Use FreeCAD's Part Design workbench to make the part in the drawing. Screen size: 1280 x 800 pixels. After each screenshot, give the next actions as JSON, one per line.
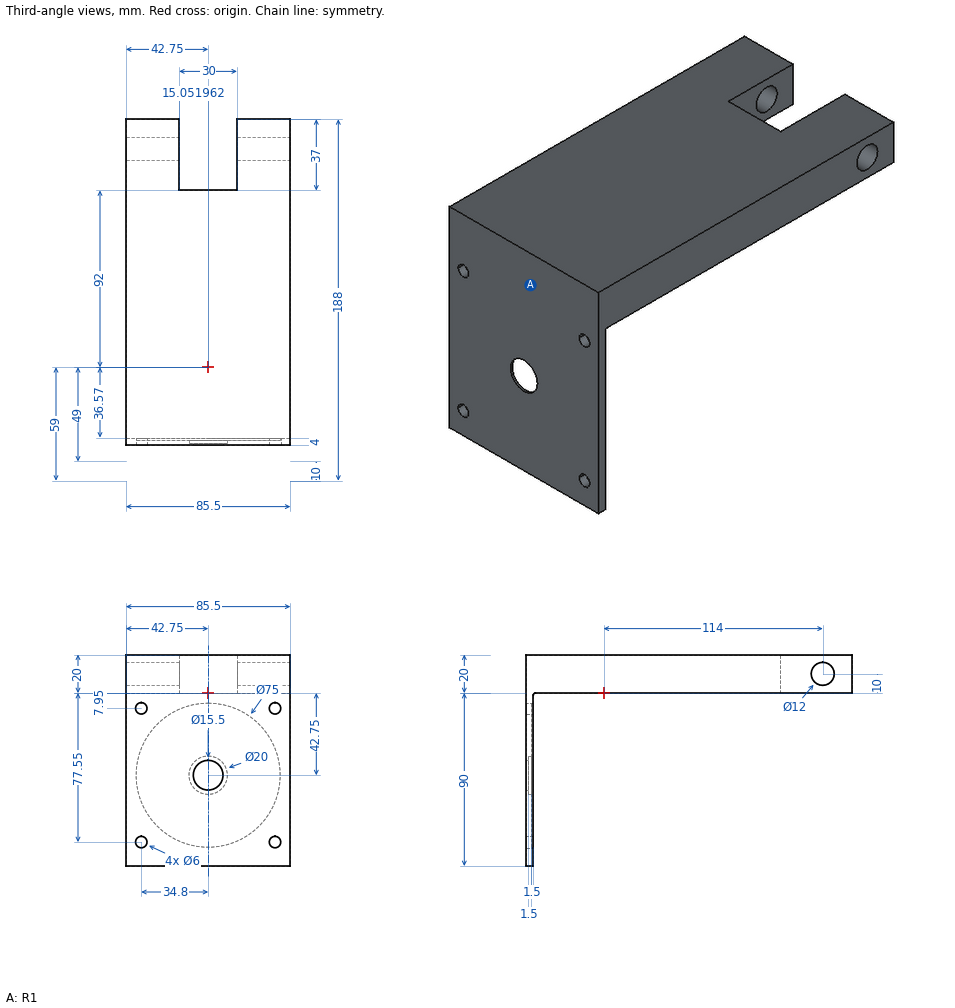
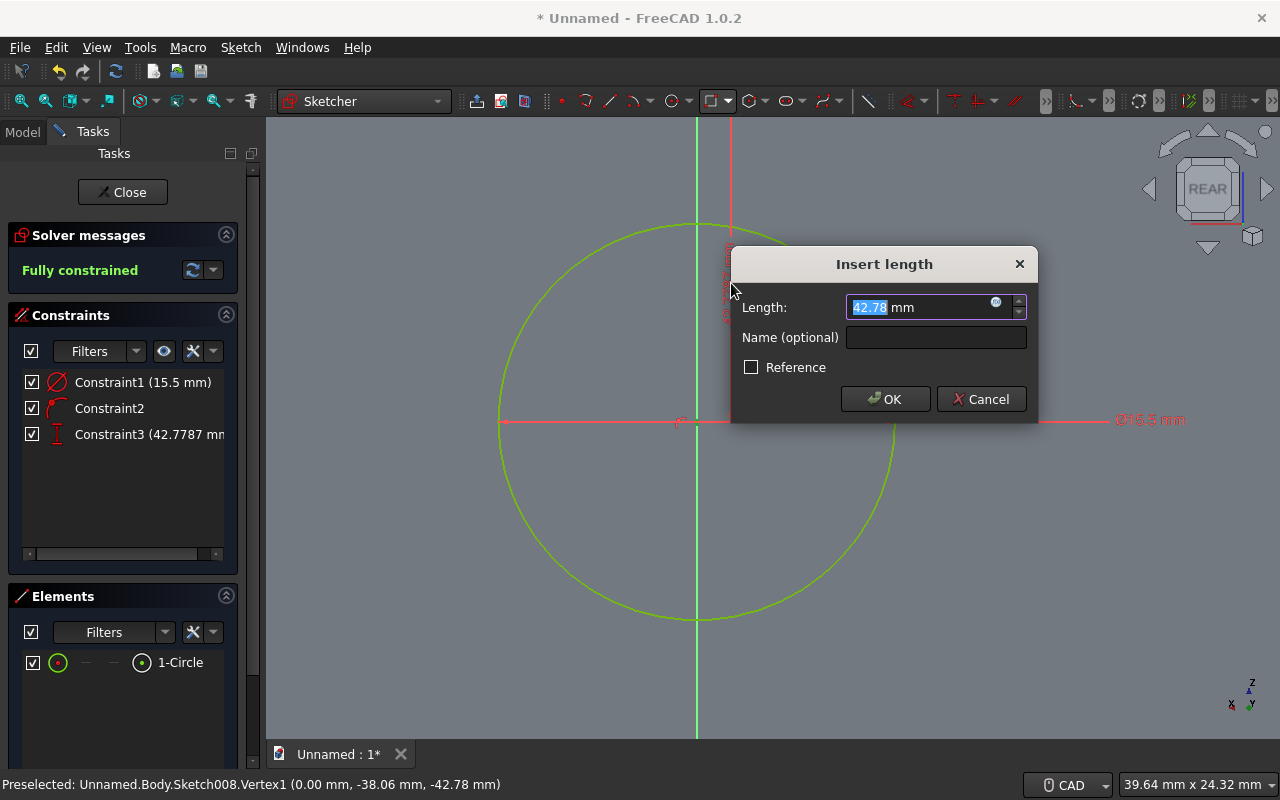
{"action": "type", "text": "42.75"}
{"action": "key", "text": "Return"}
{"action": "key", "text": "Escape"}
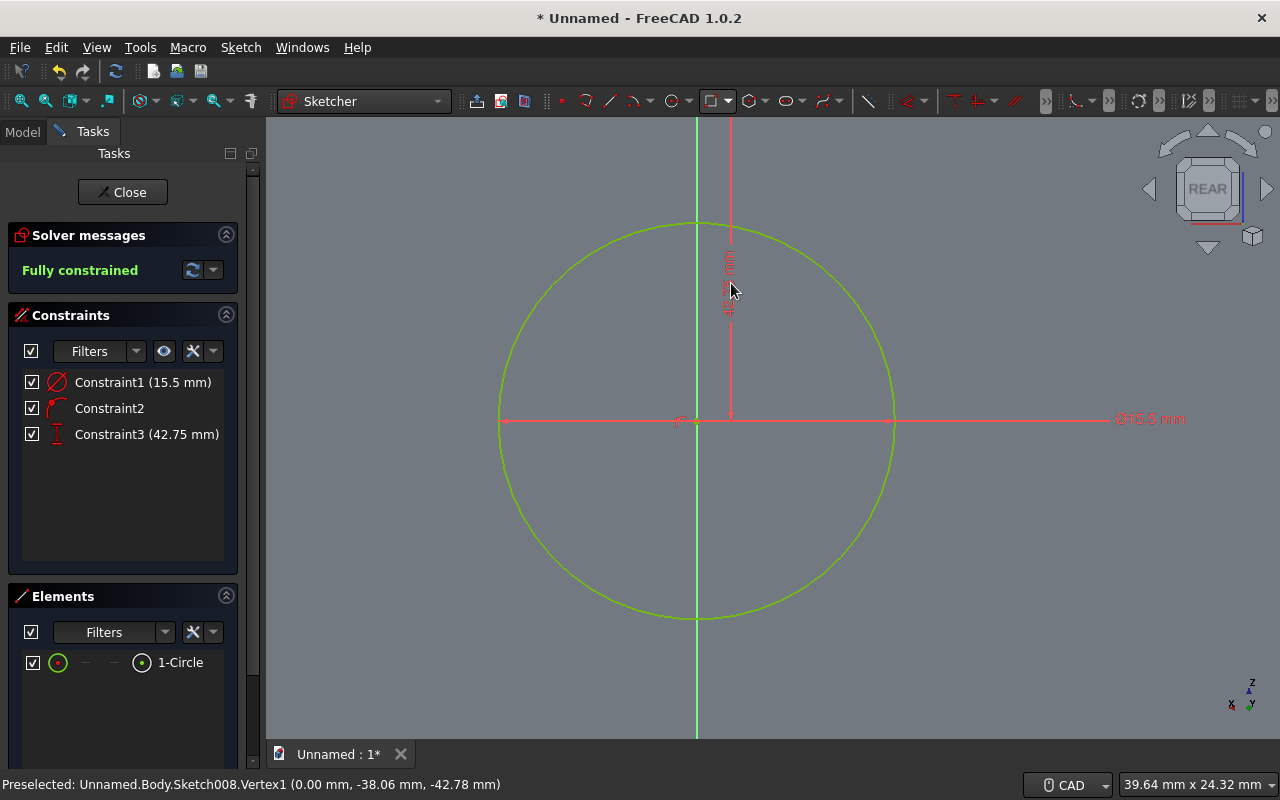
{"action": "left_click", "coordinate": [123, 192]}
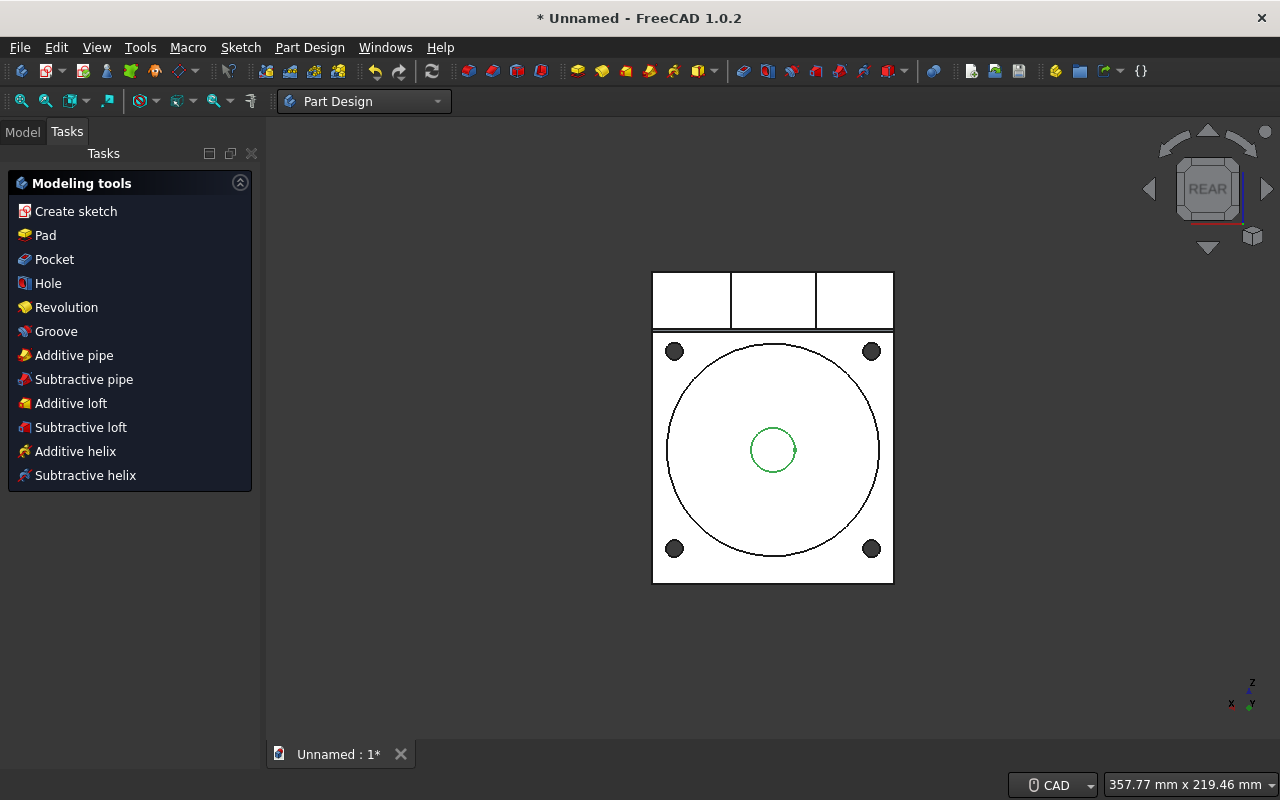
{"action": "left_click", "coordinate": [744, 72]}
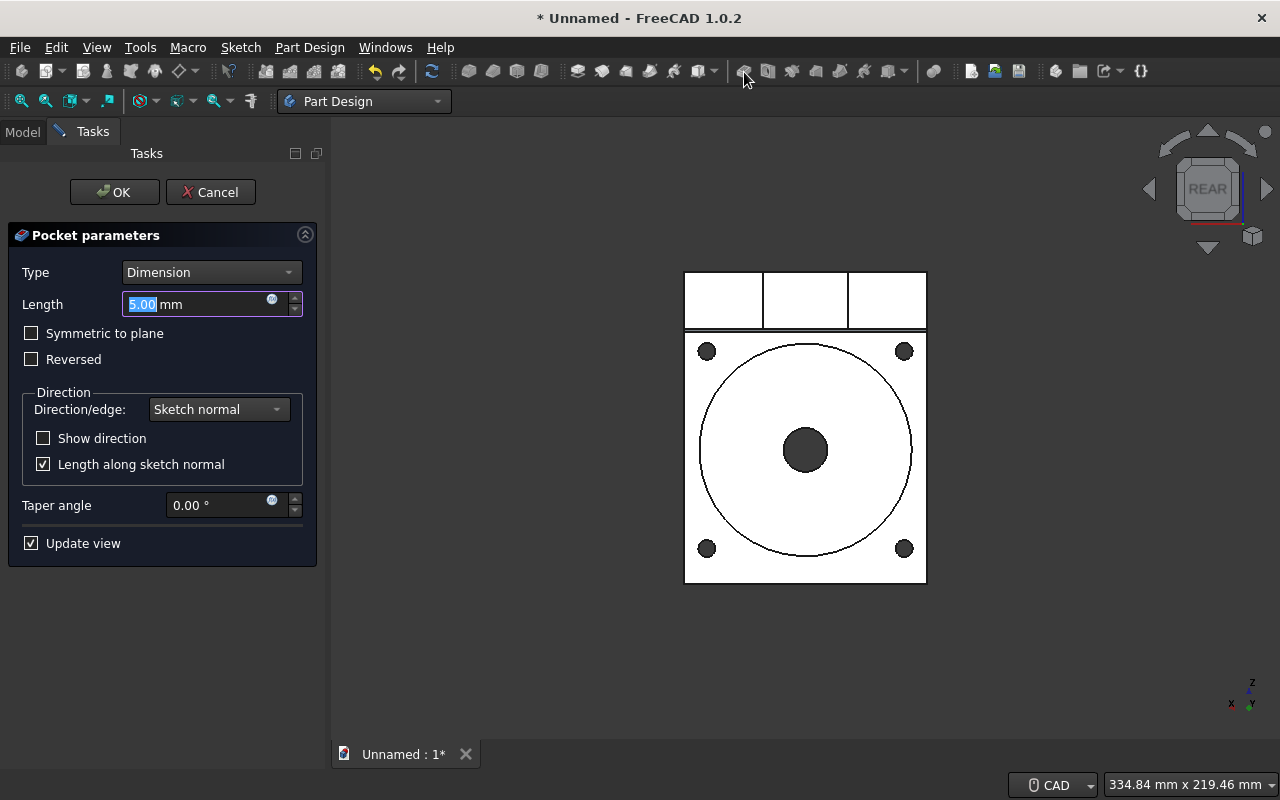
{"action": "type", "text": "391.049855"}
{"action": "key", "text": "Tab"}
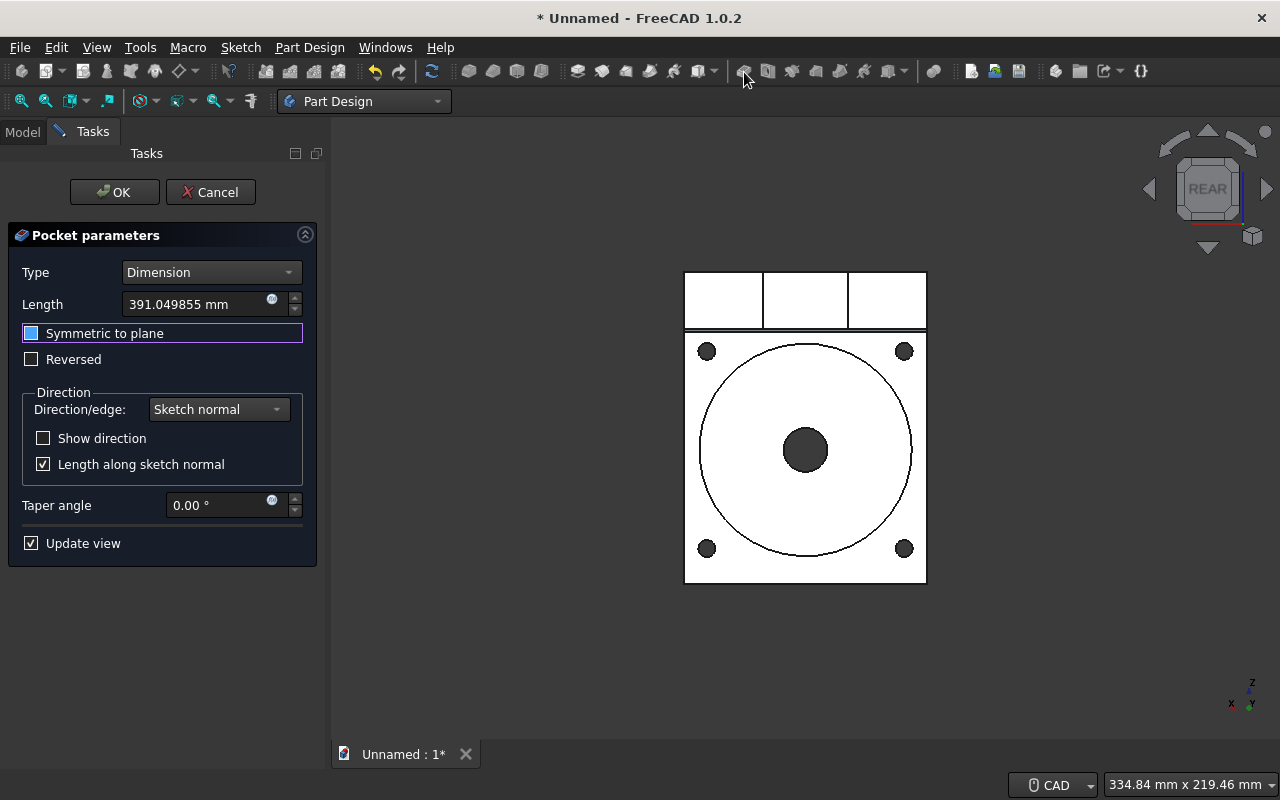
{"action": "left_click", "coordinate": [30, 333]}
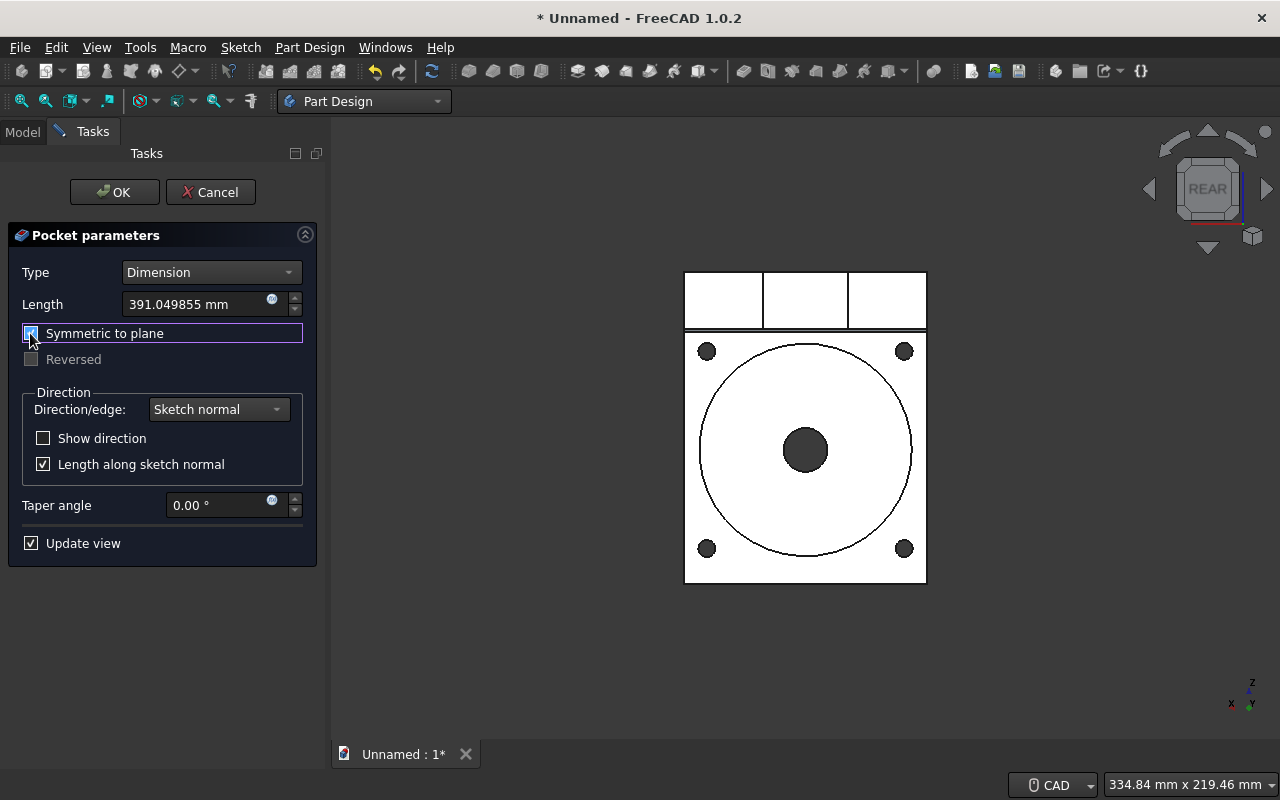
{"action": "left_click", "coordinate": [115, 192]}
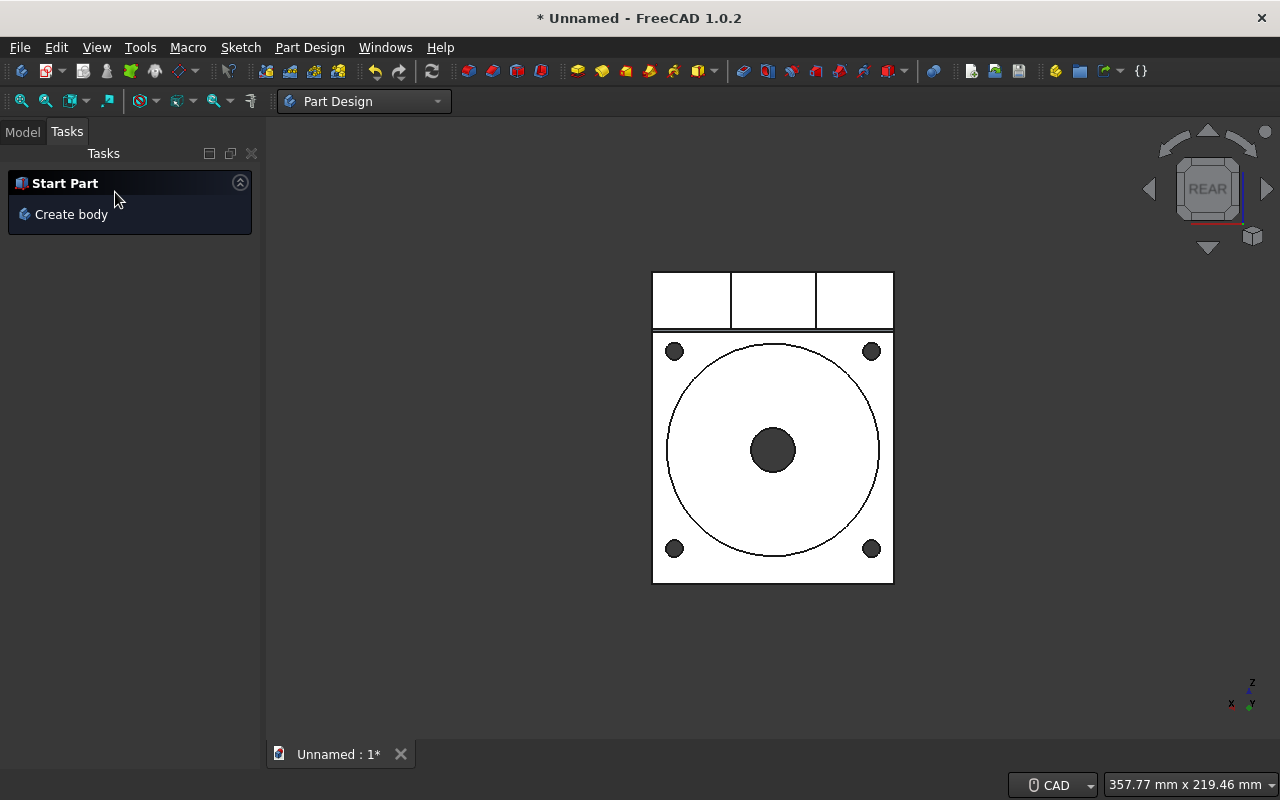
{"action": "left_click", "coordinate": [712, 449]}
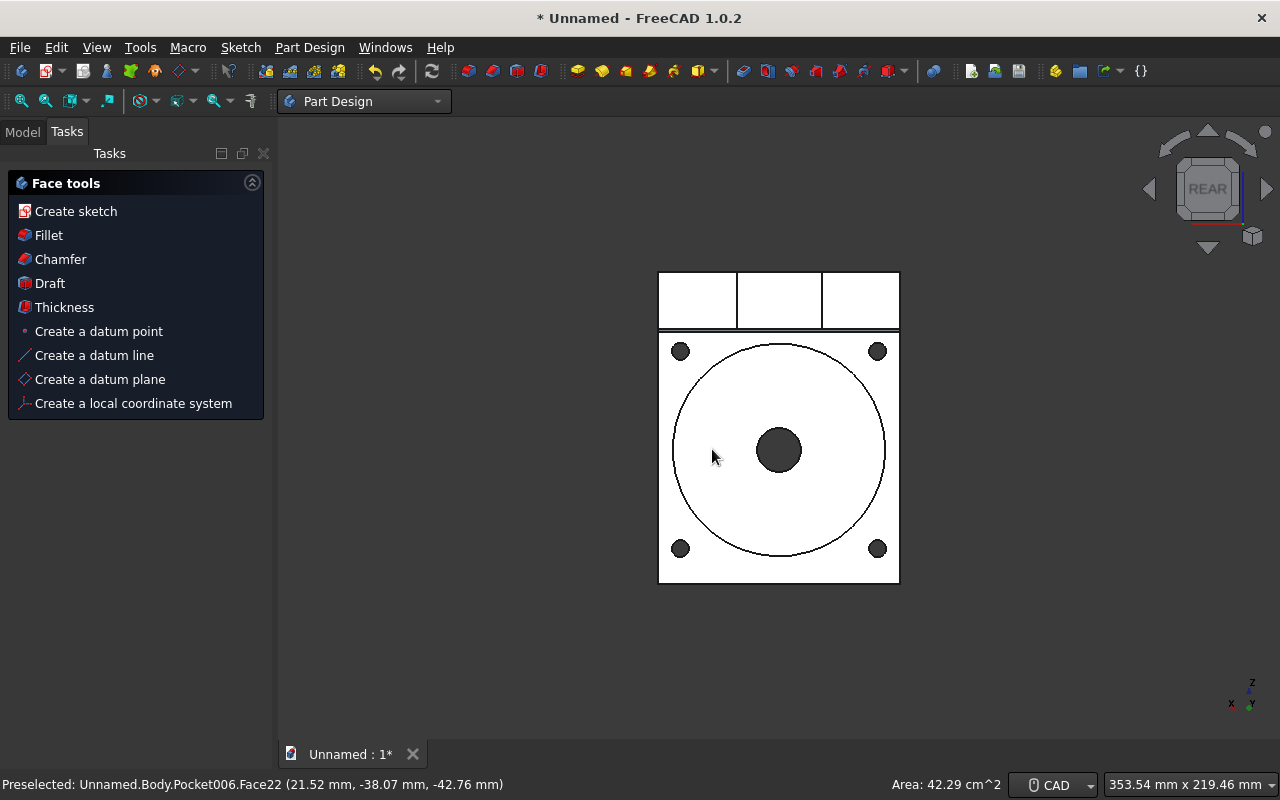
{"action": "left_click", "coordinate": [46, 72]}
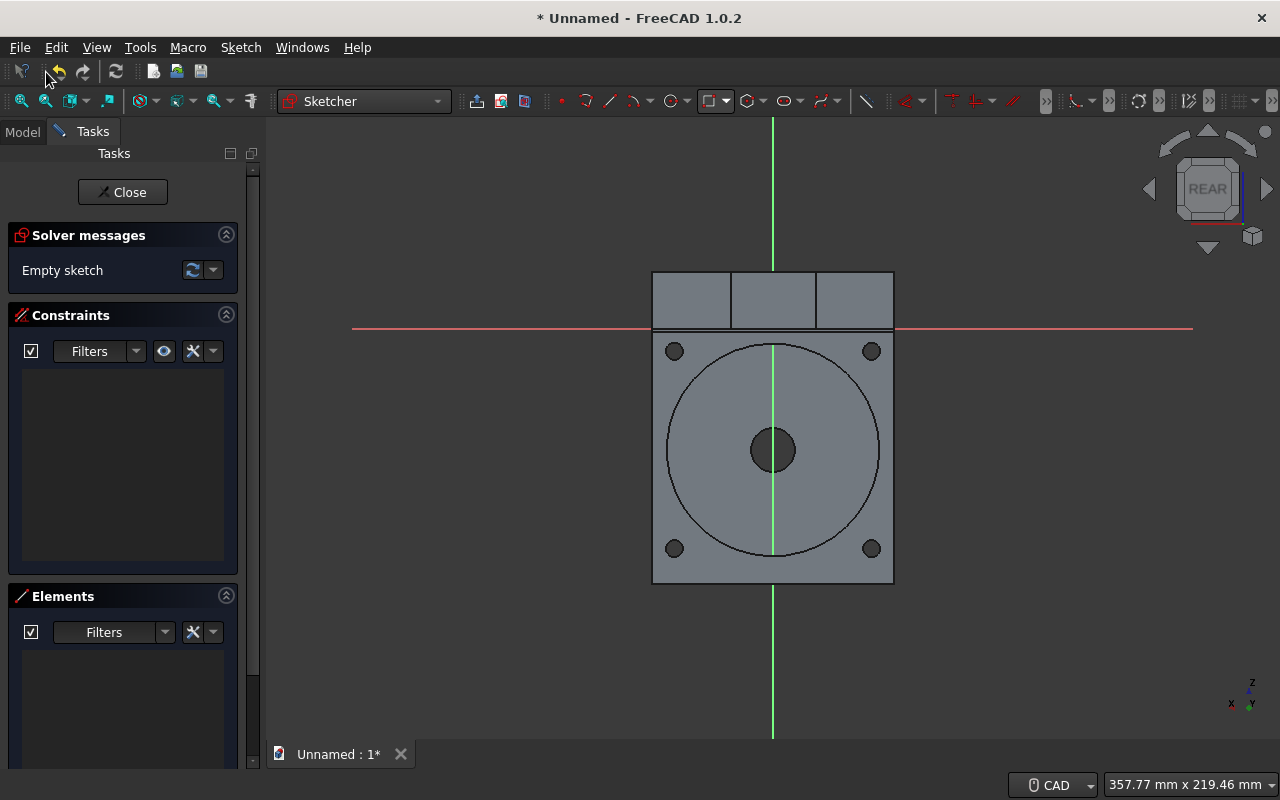
{"action": "left_click", "coordinate": [526, 102]}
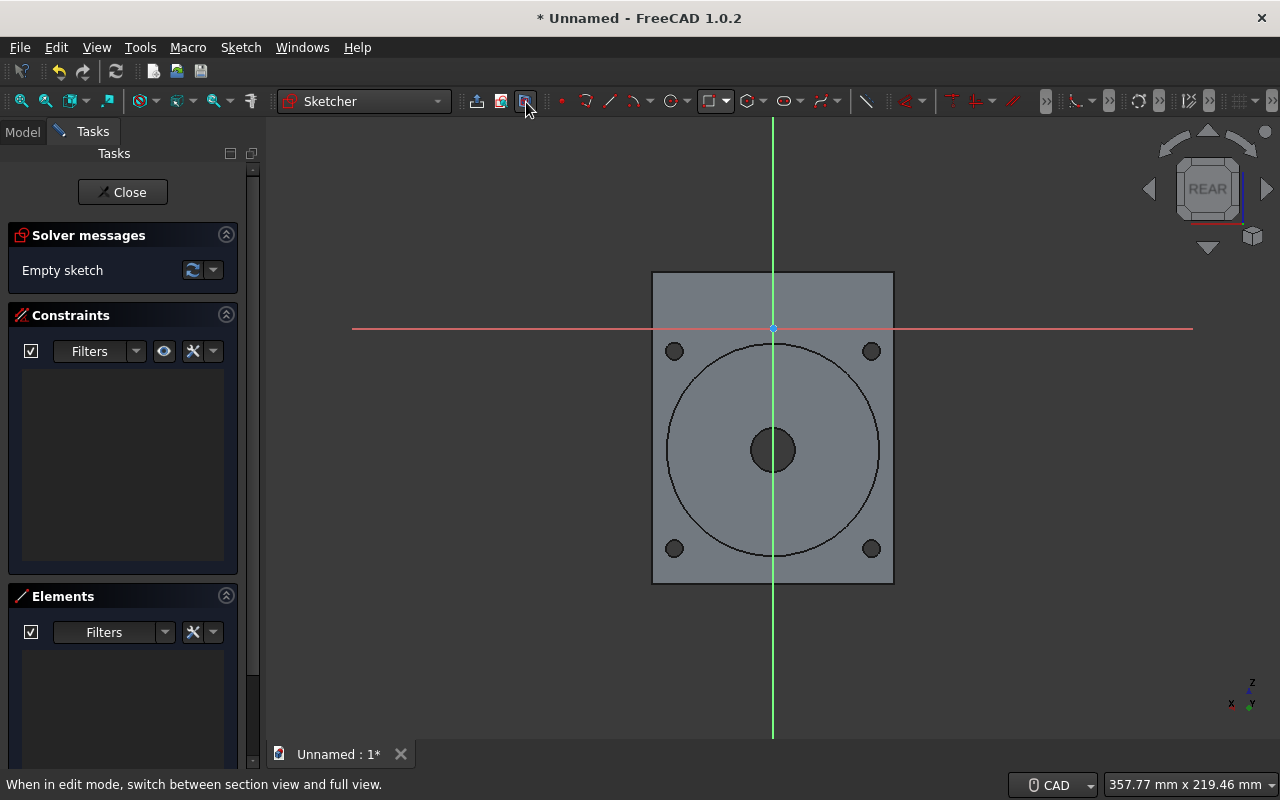
{"action": "scroll", "coordinate": [784, 453], "scroll_direction": "up", "scroll_amount": 10}